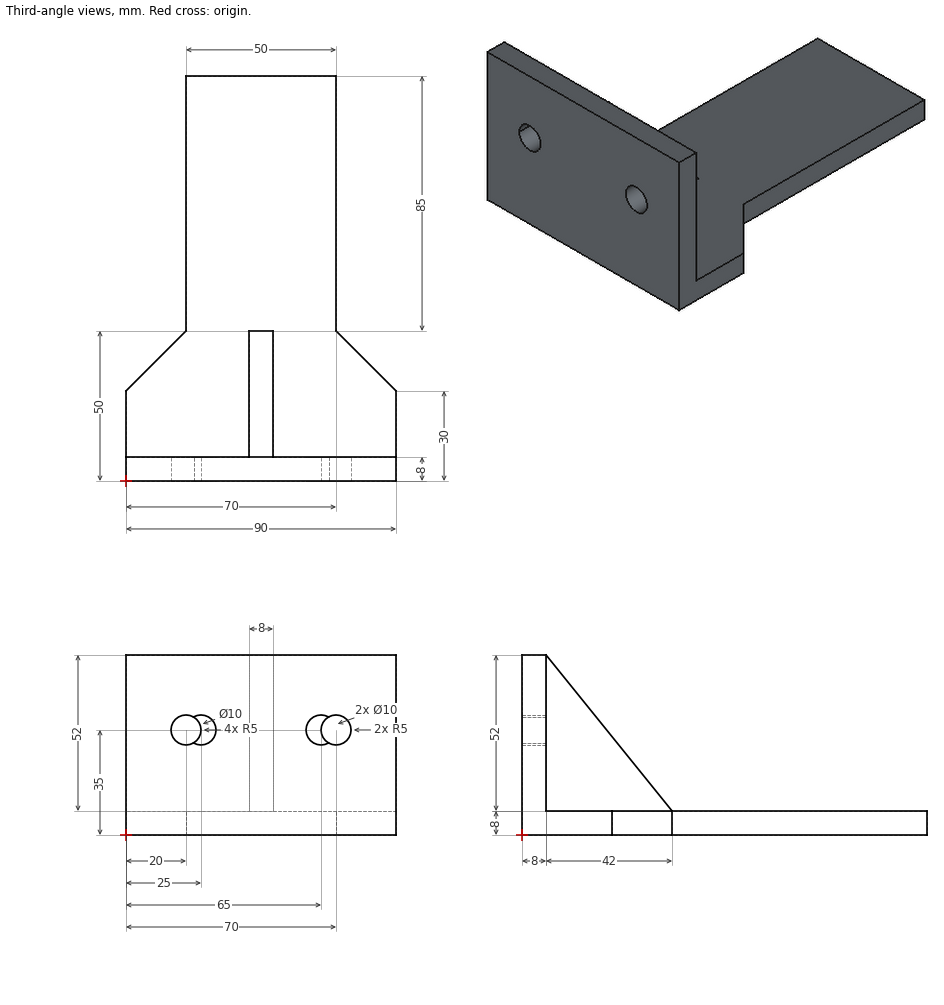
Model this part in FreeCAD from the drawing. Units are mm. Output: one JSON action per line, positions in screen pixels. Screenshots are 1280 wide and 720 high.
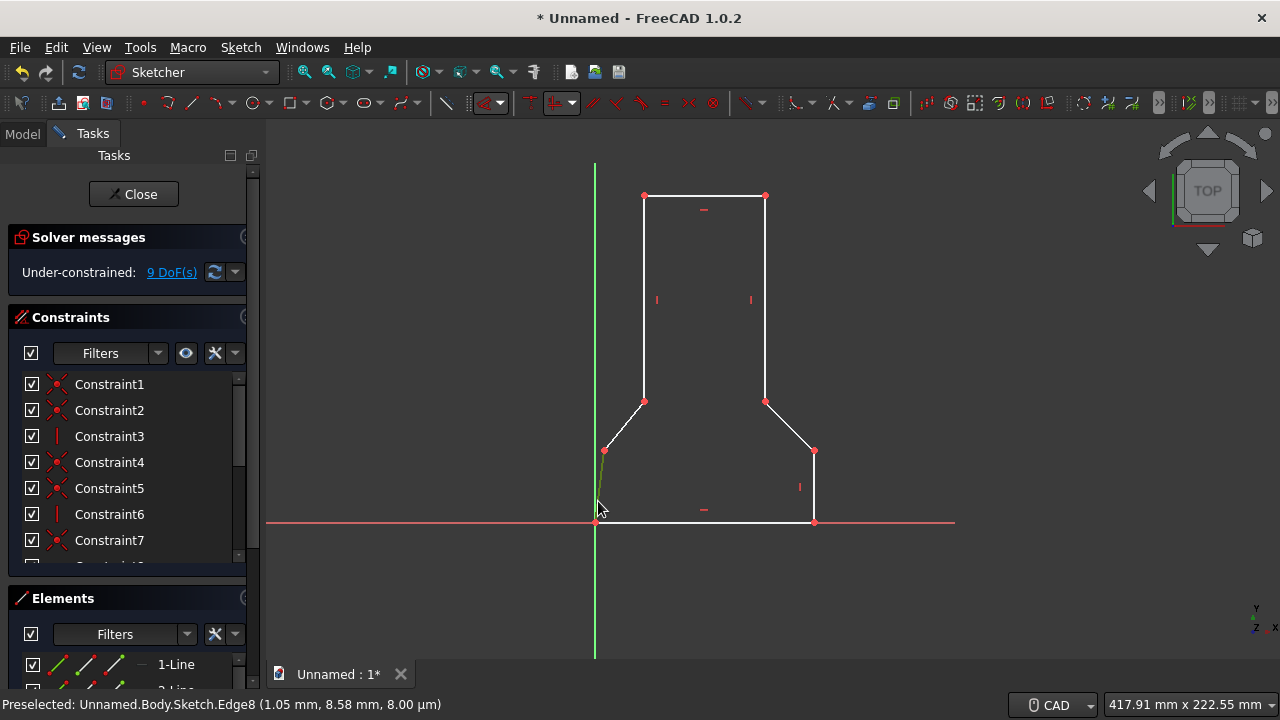
{"action": "left_click", "coordinate": [574, 104]}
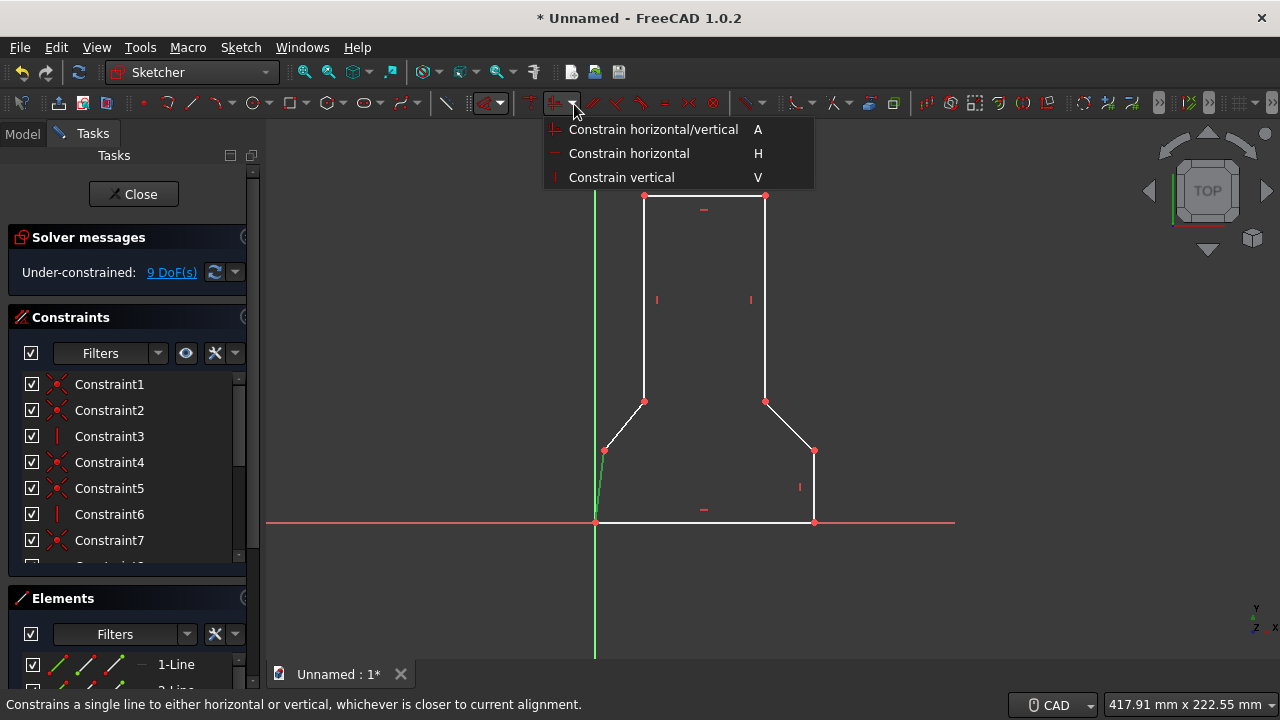
{"action": "left_click", "coordinate": [679, 177]}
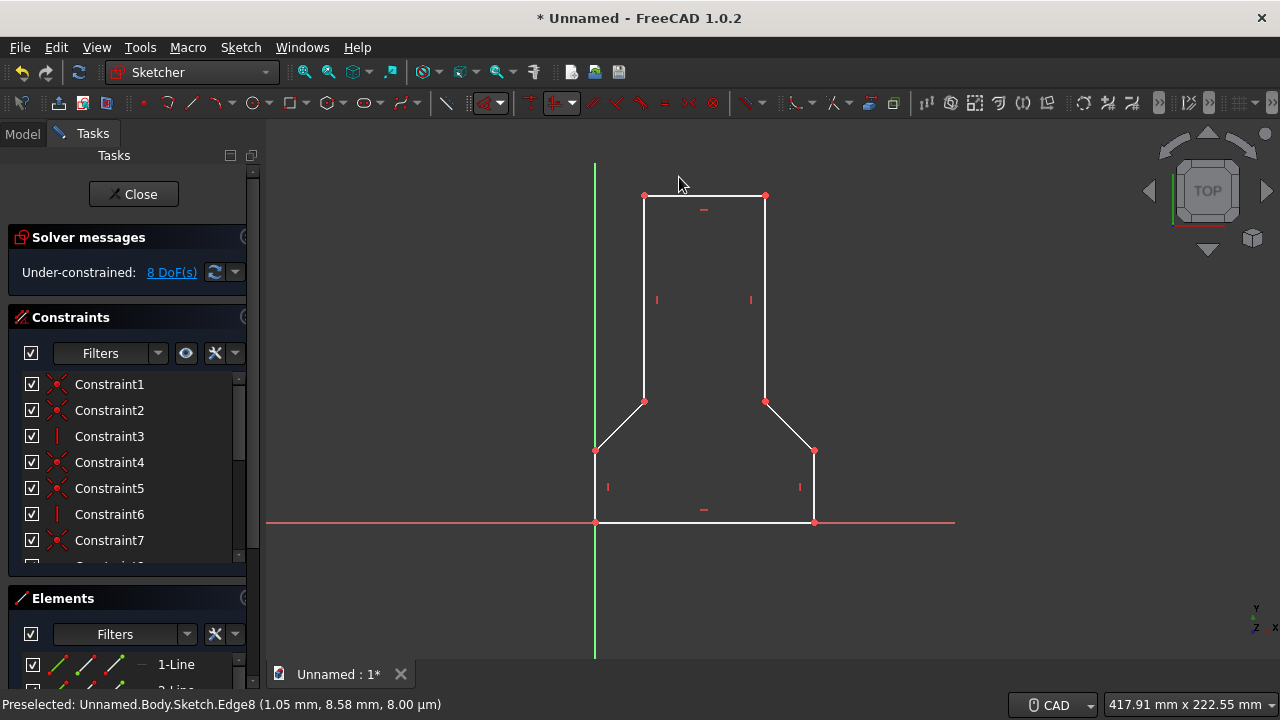
{"action": "left_click", "coordinate": [484, 104]}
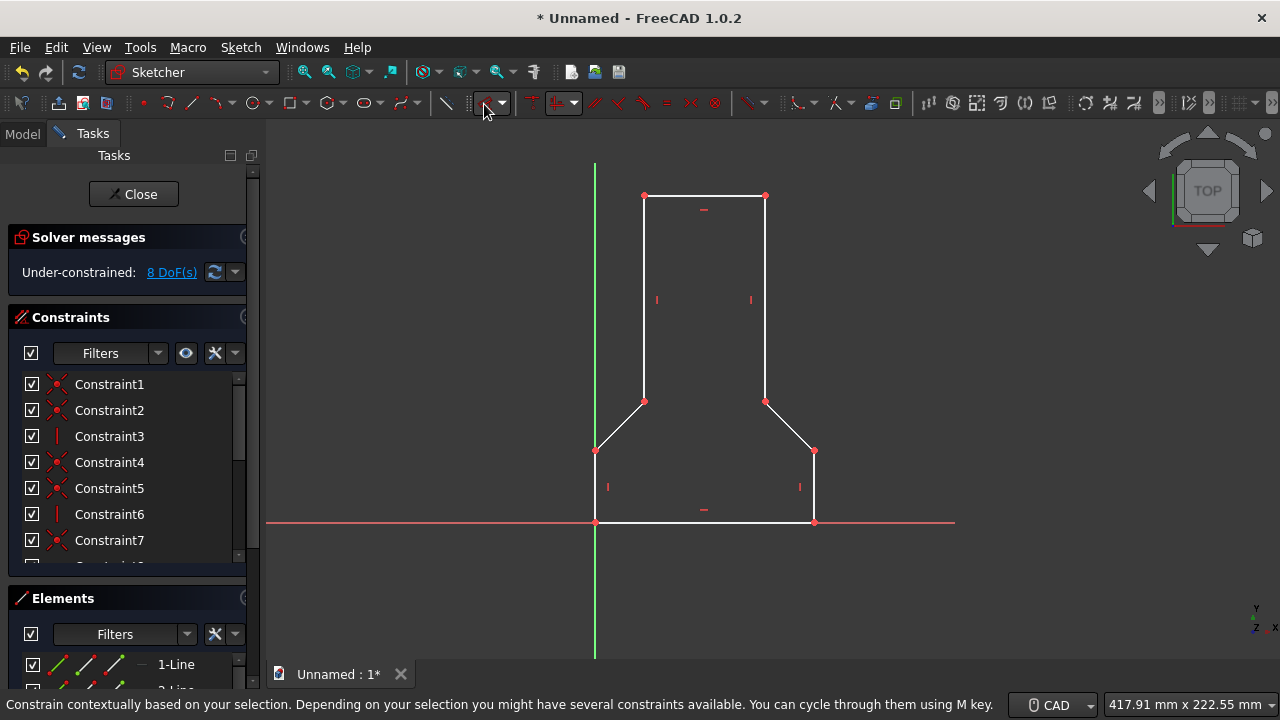
{"action": "left_click", "coordinate": [661, 523]}
{"action": "left_click", "coordinate": [705, 557]}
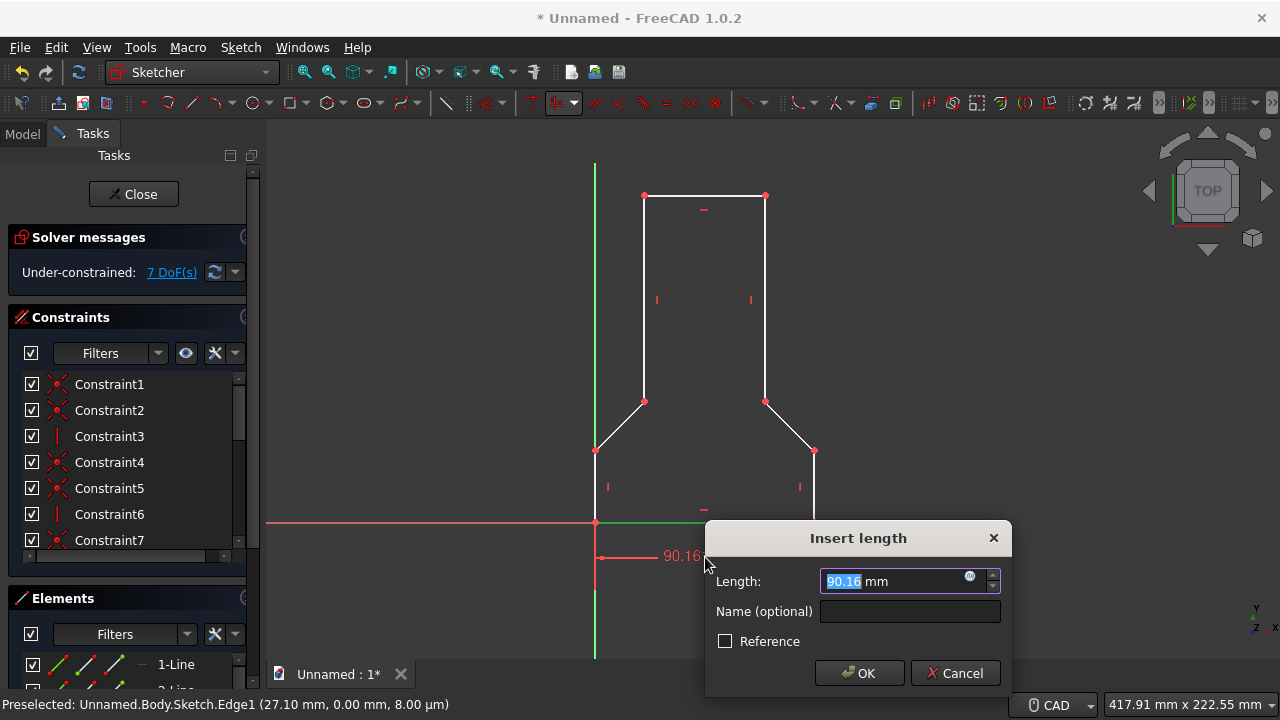
{"action": "type", "text": "90"}
{"action": "key", "text": "Return"}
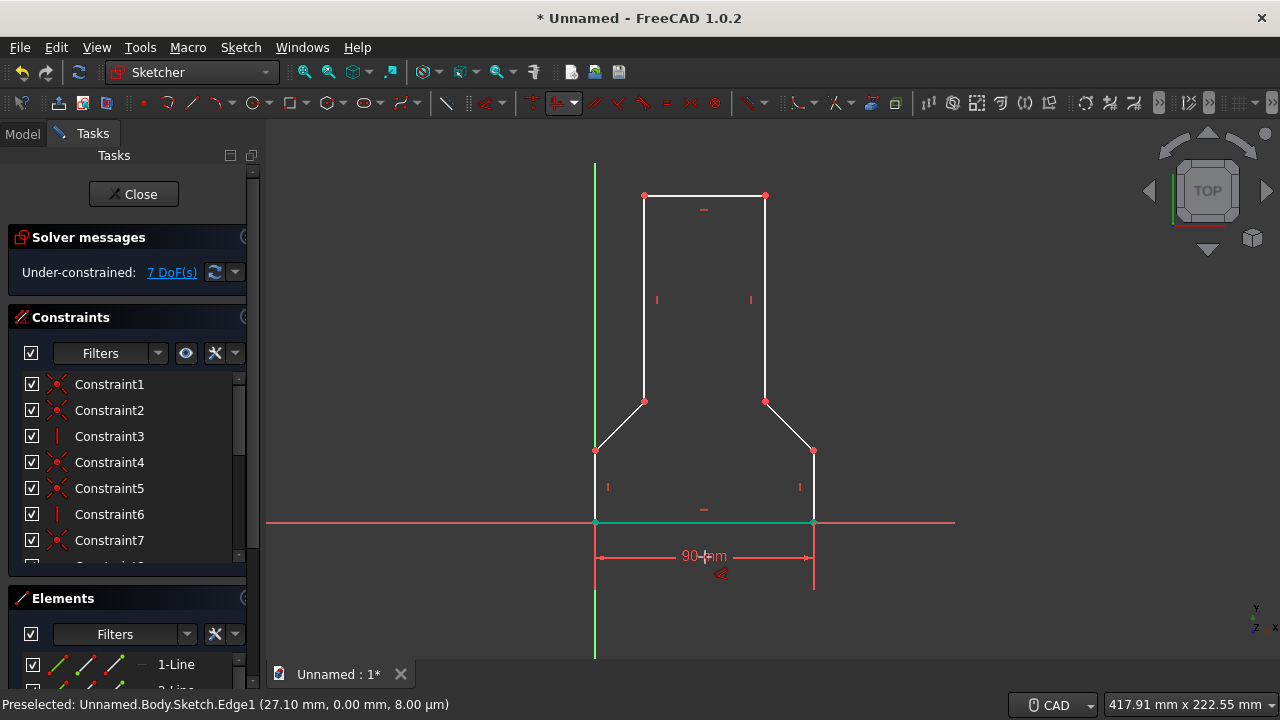
{"action": "left_click", "coordinate": [814, 501]}
{"action": "left_click", "coordinate": [848, 487]}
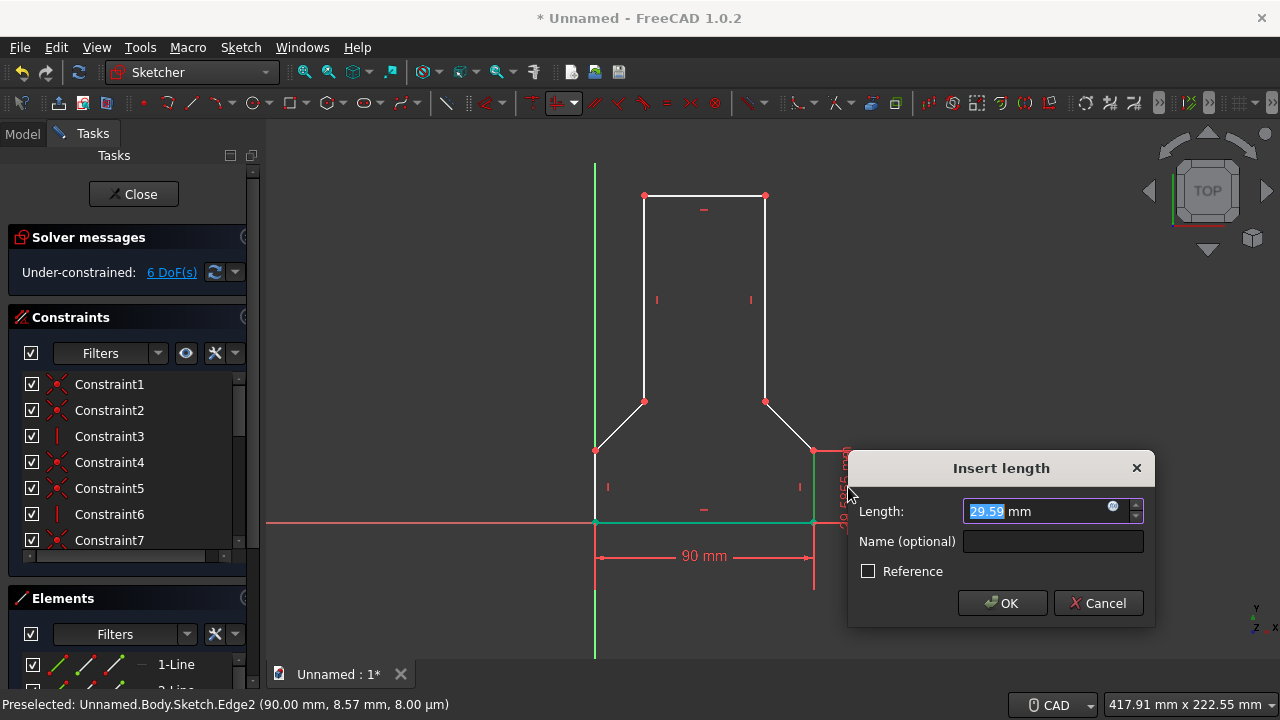
{"action": "type", "text": "30"}
{"action": "key", "text": "Return"}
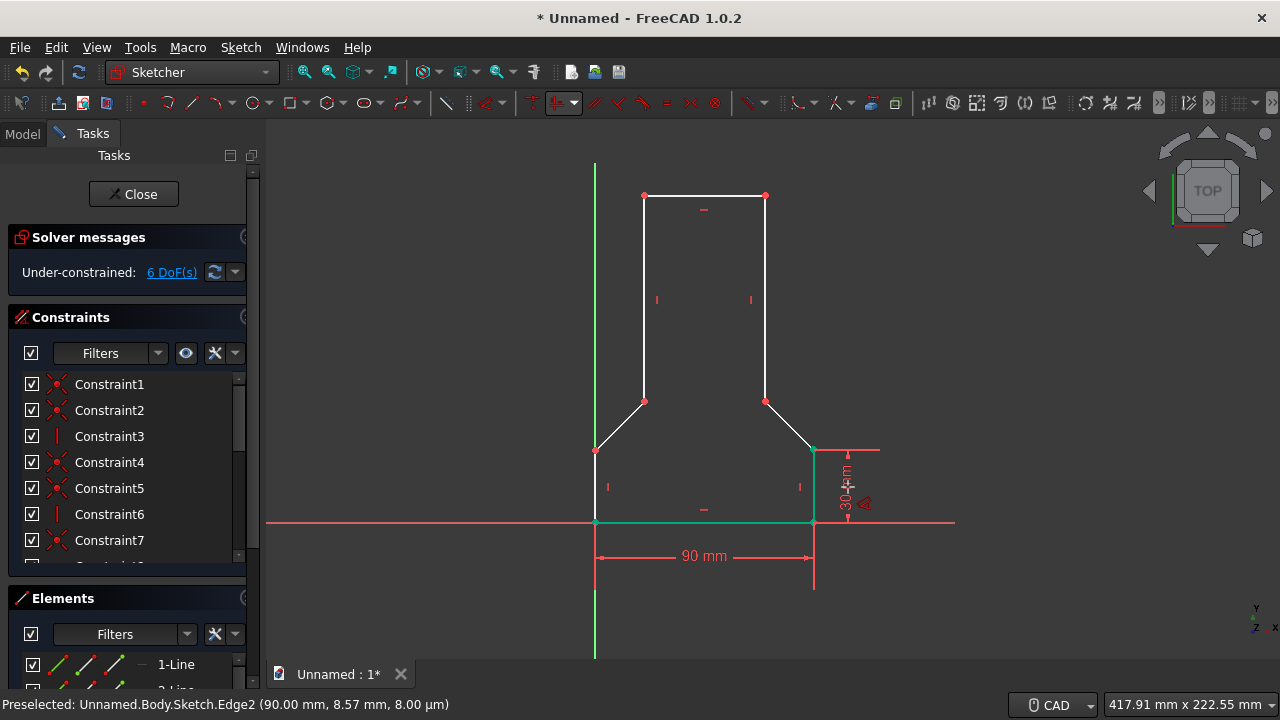
{"action": "left_click", "coordinate": [765, 340]}
{"action": "left_click", "coordinate": [799, 299]}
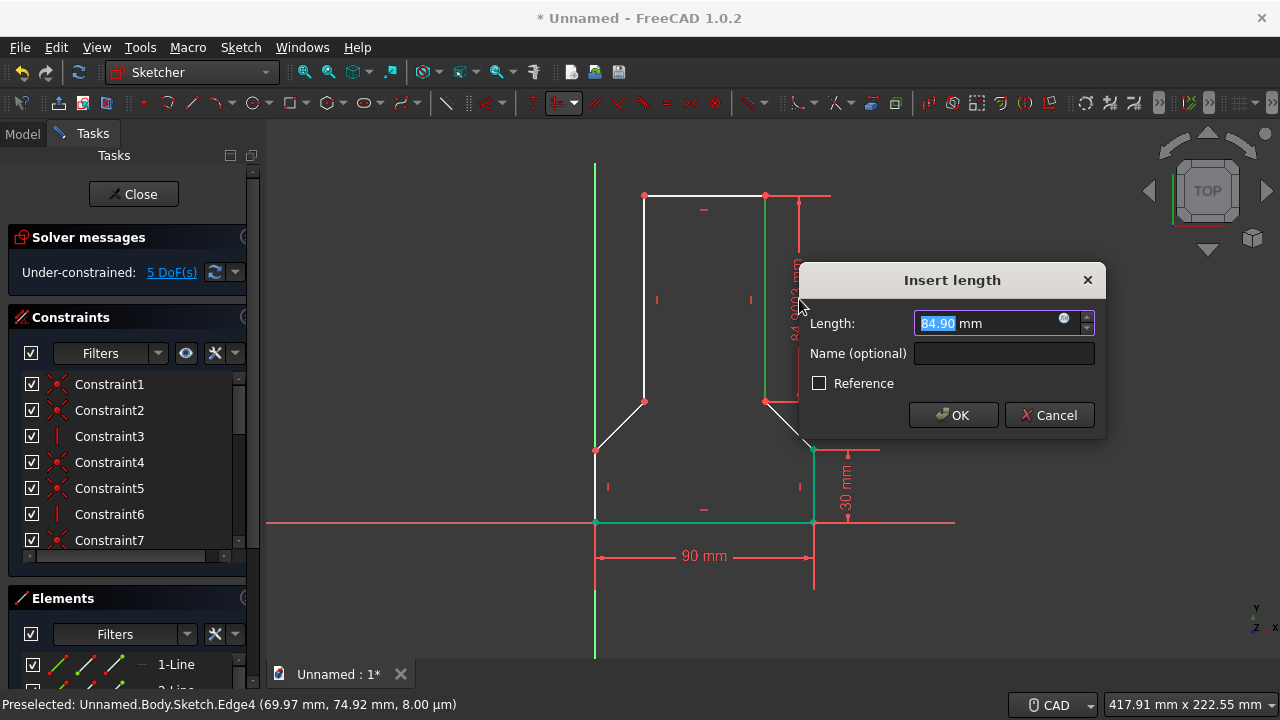
{"action": "type", "text": "85"}
{"action": "key", "text": "Return"}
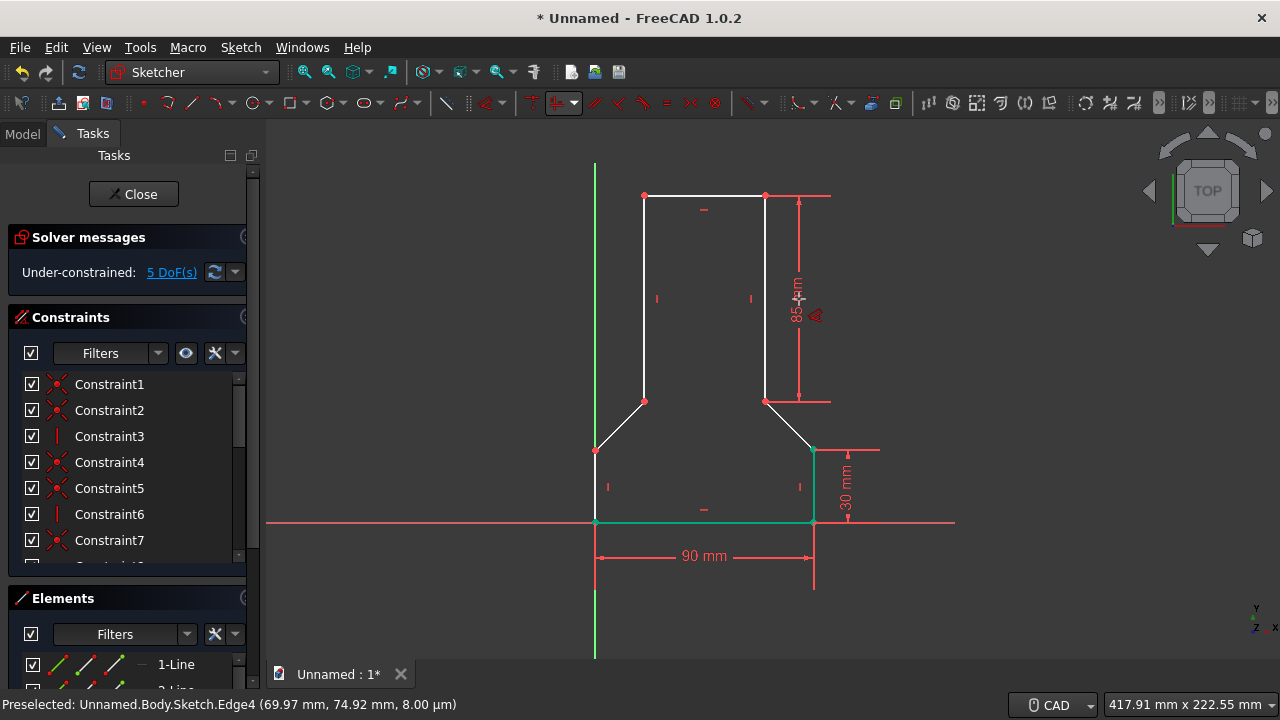
{"action": "left_click", "coordinate": [729, 196]}
{"action": "left_click", "coordinate": [705, 162]}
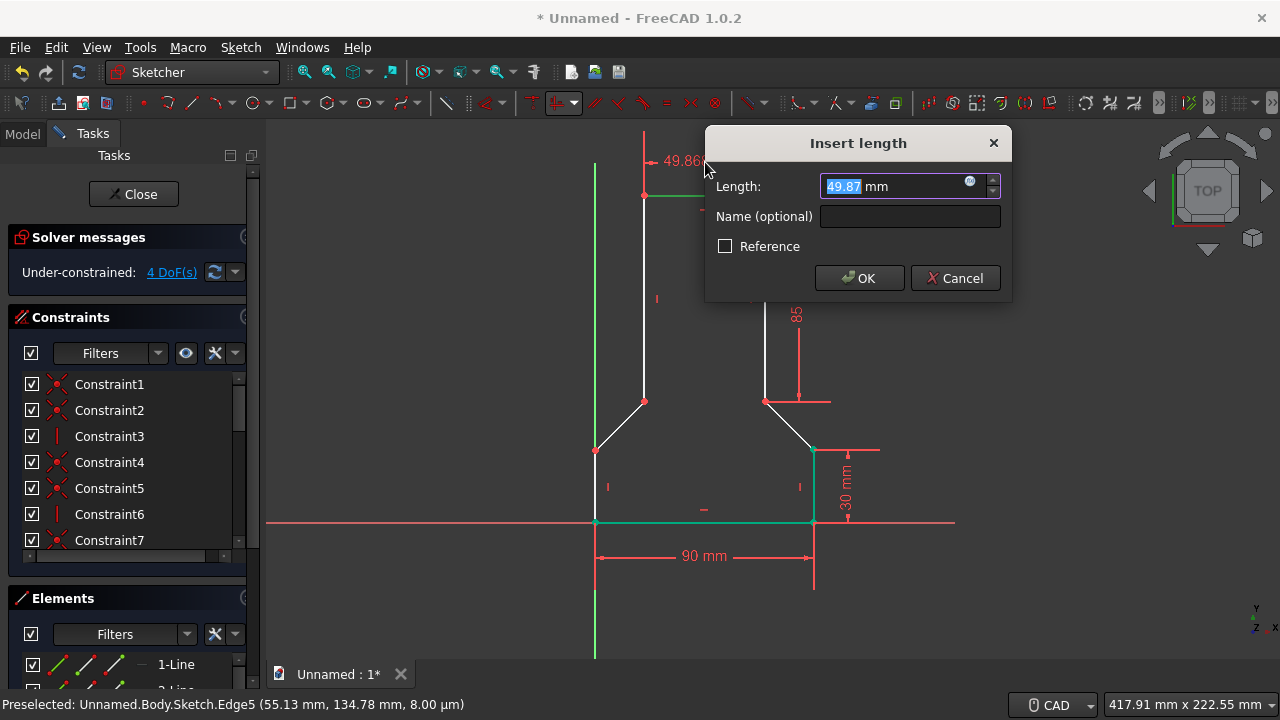
{"action": "type", "text": "50"}
{"action": "key", "text": "Return"}